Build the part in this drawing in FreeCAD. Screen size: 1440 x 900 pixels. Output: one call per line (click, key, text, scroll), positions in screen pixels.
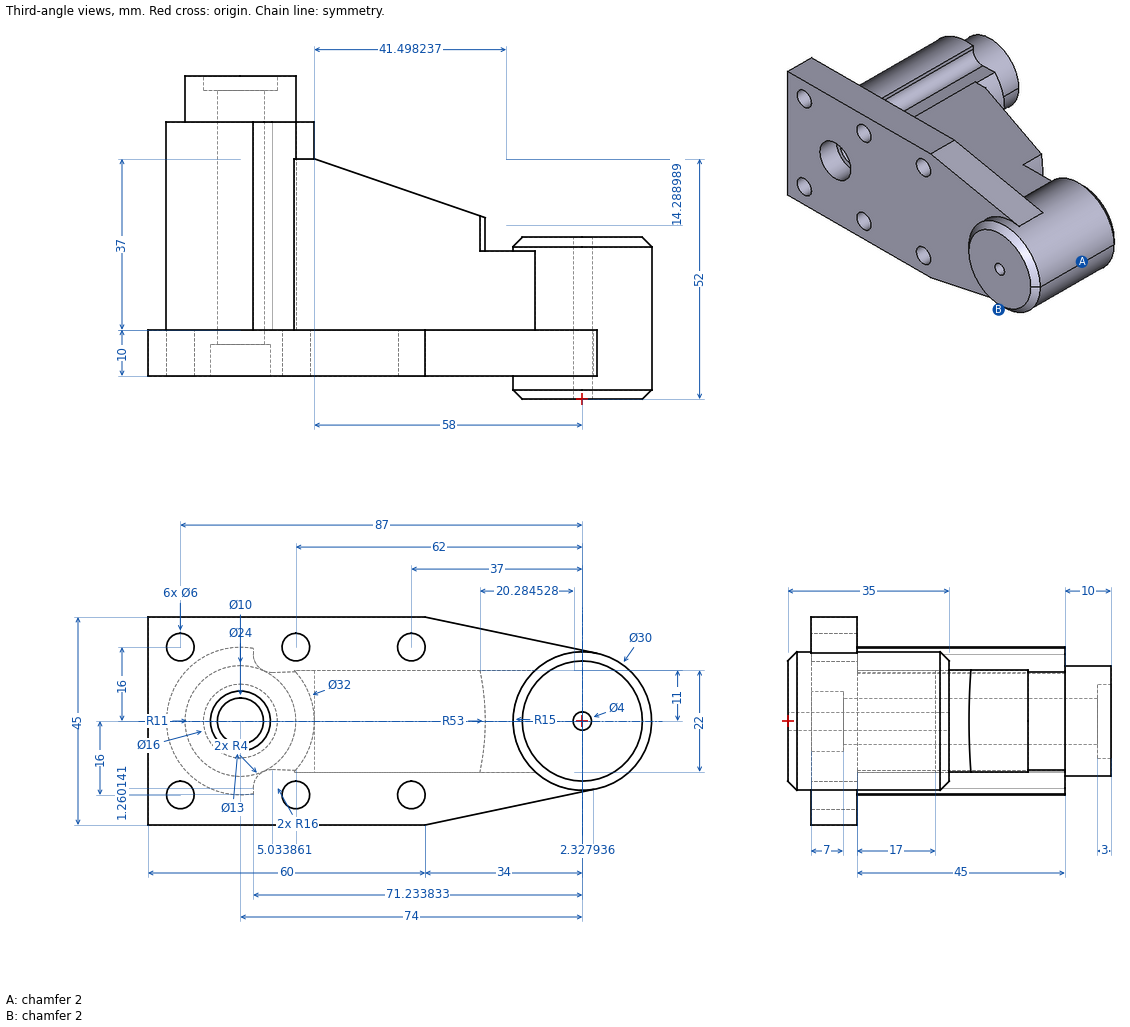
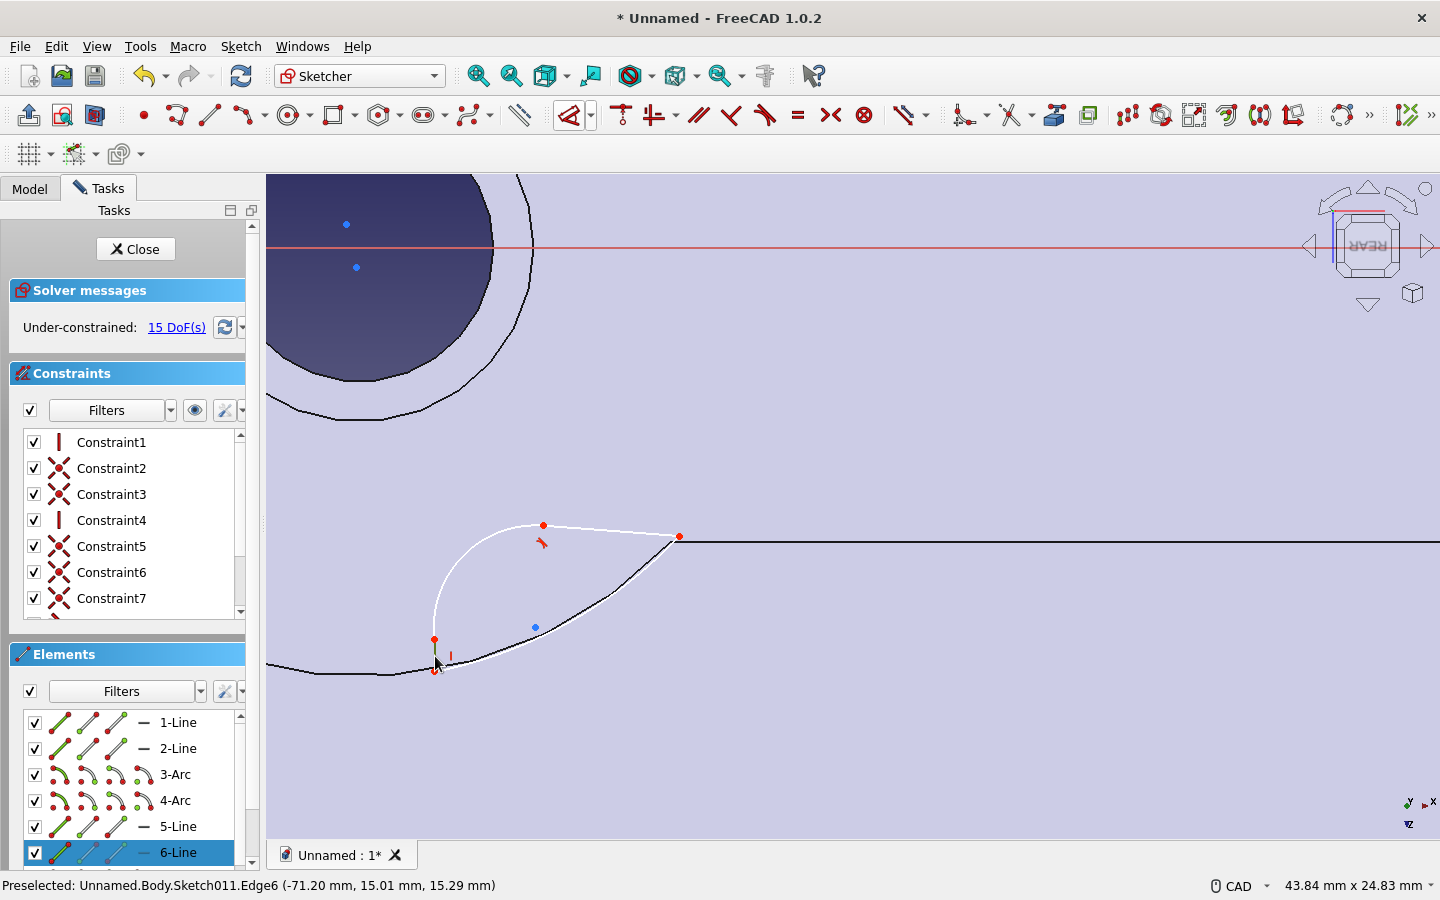
click(491, 536)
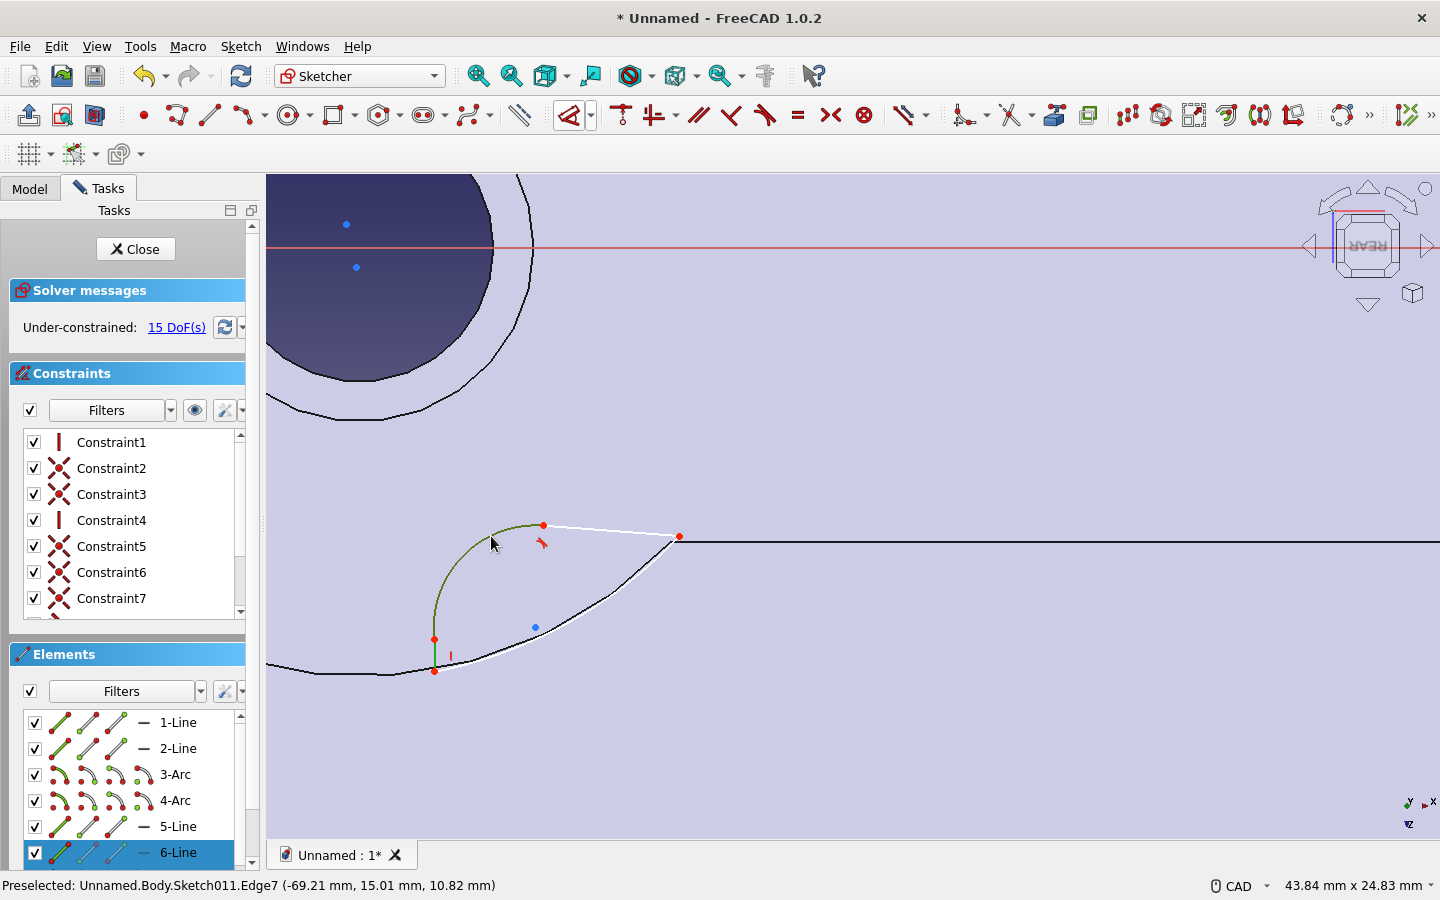
click(765, 116)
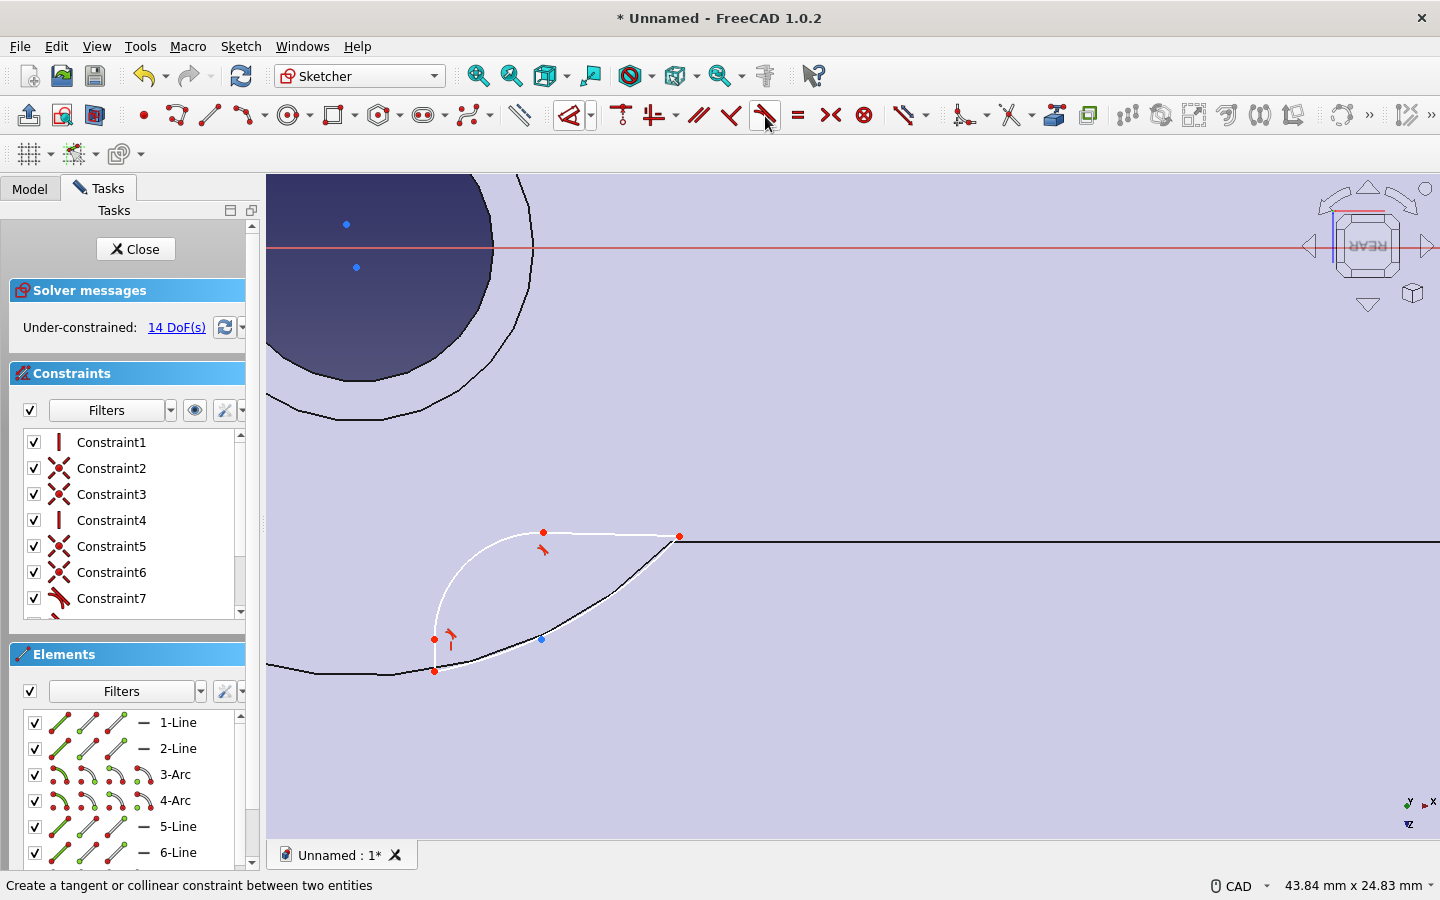
scroll(434, 657, down, 5)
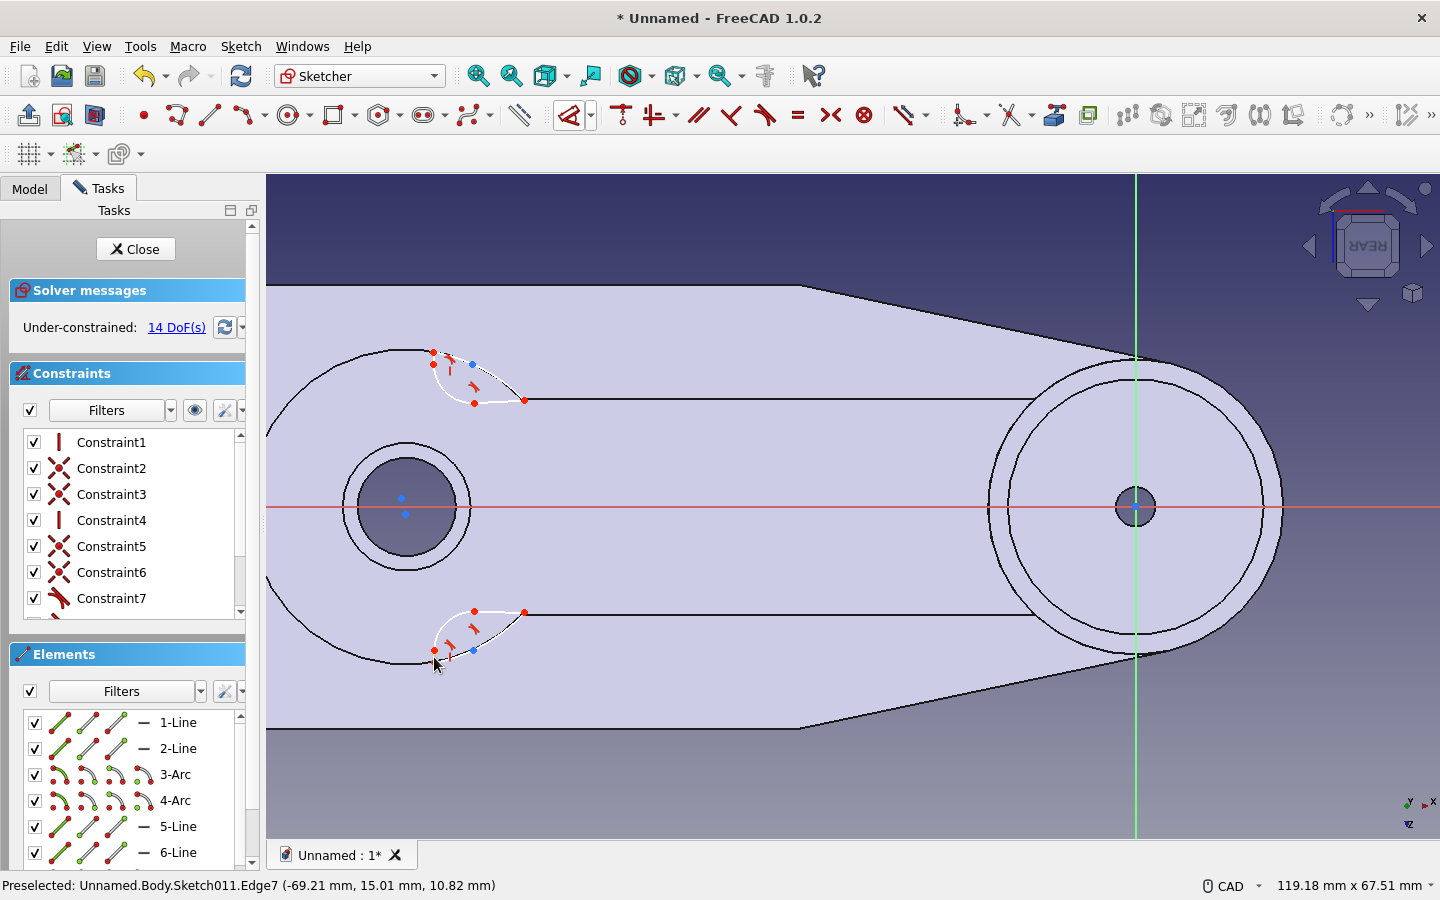
click(501, 380)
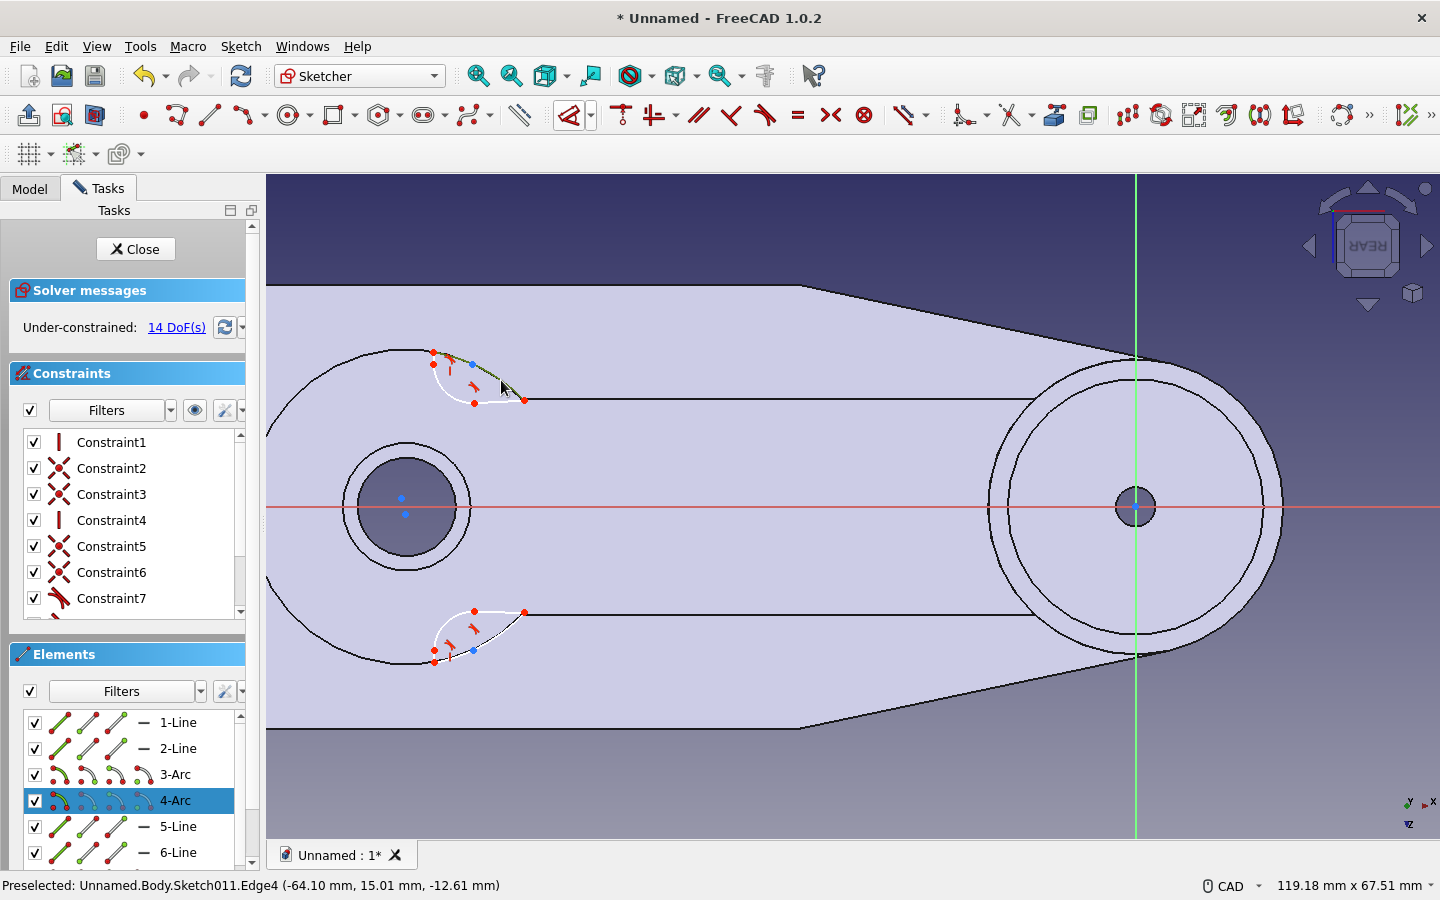
click(464, 654)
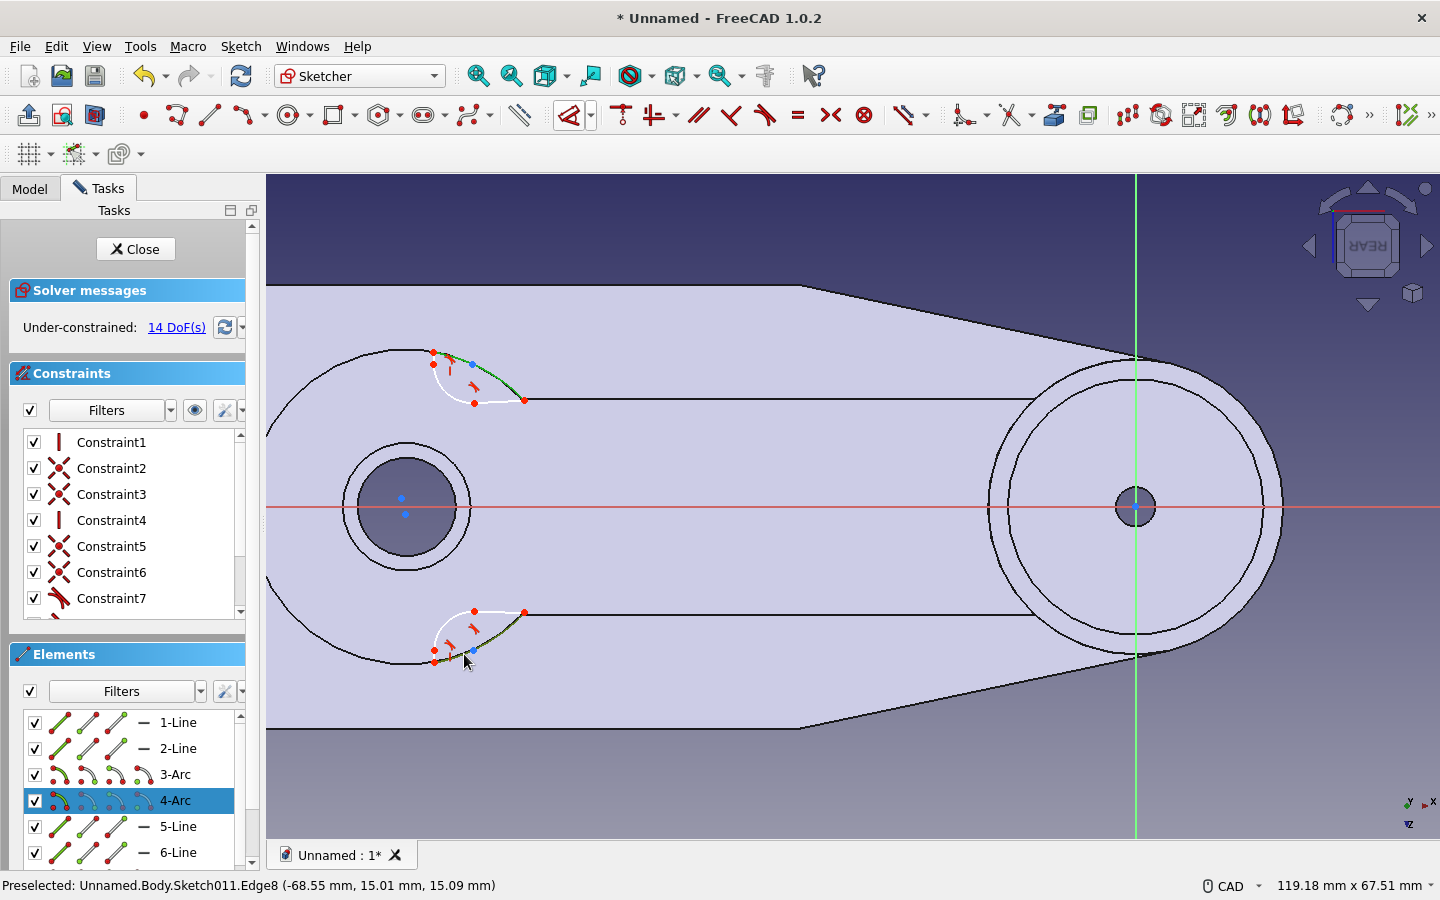
click(621, 116)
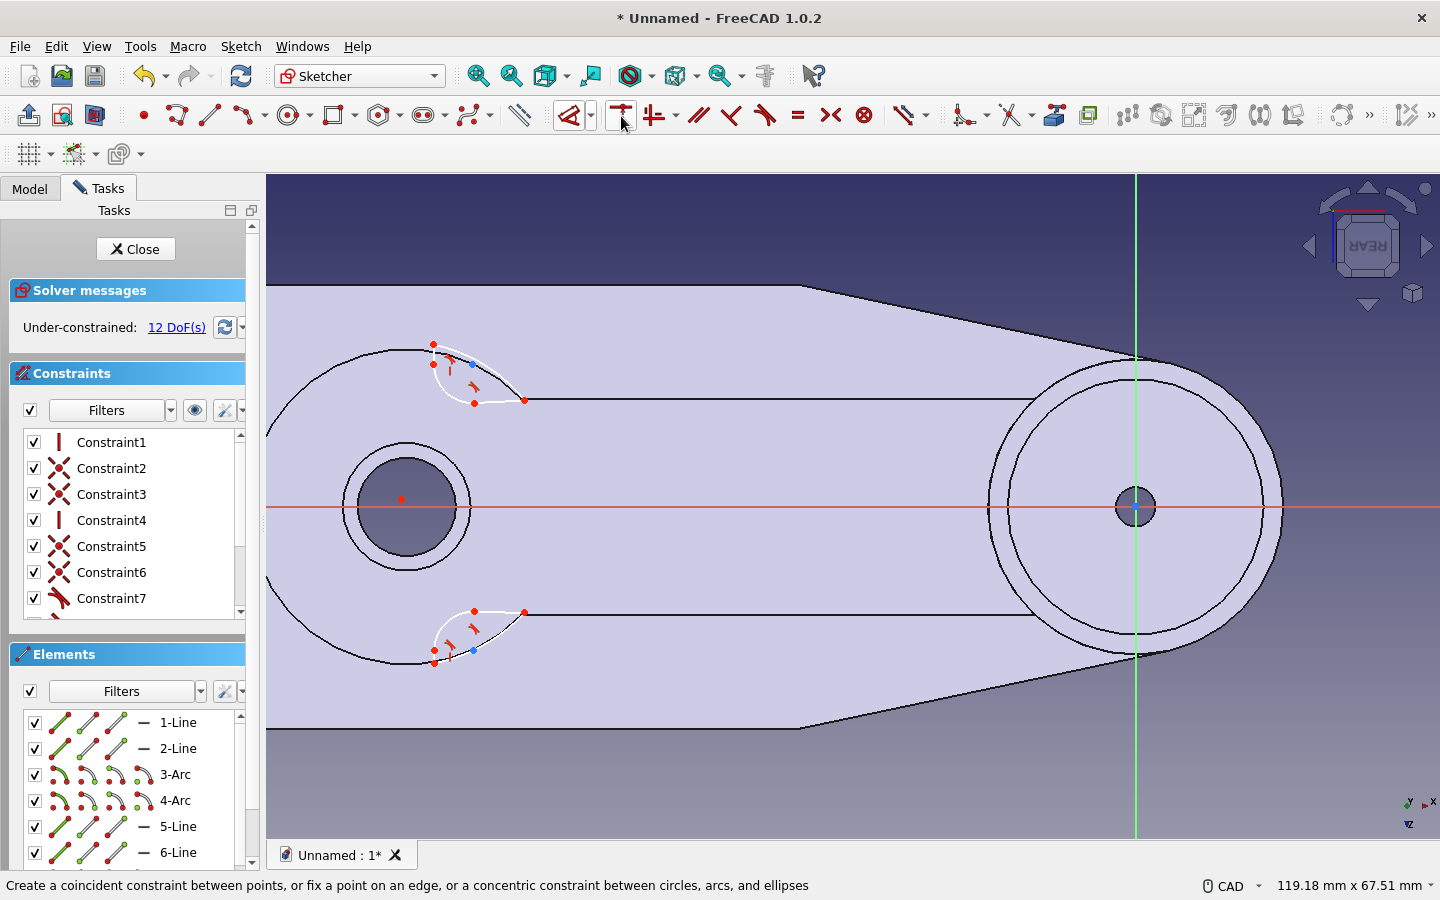
click(439, 382)